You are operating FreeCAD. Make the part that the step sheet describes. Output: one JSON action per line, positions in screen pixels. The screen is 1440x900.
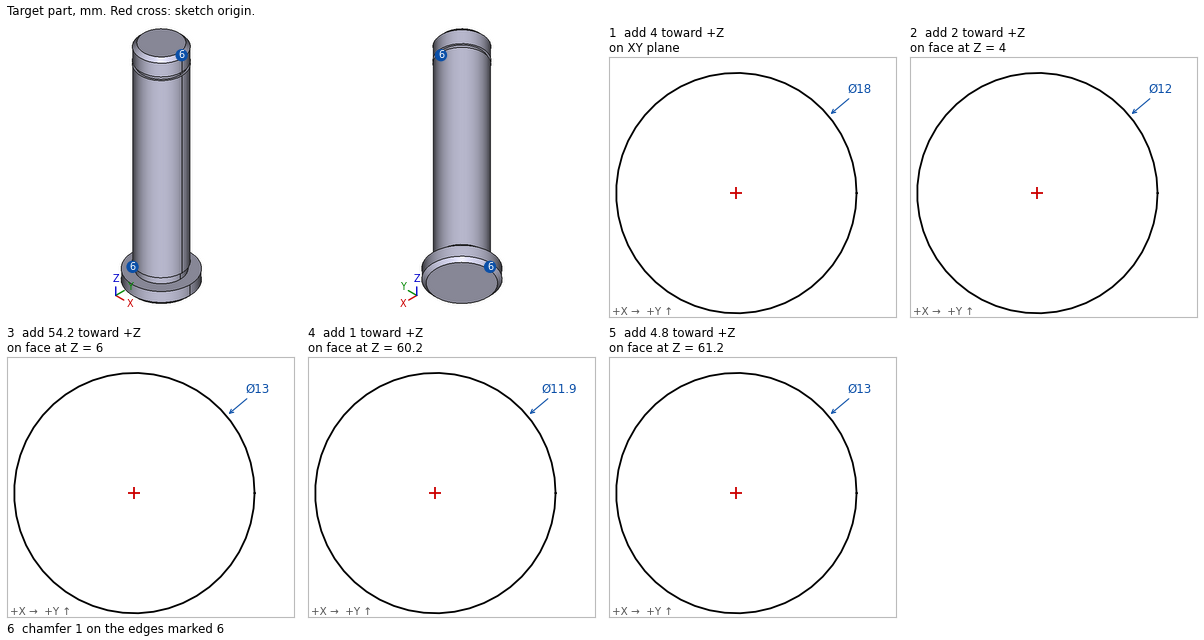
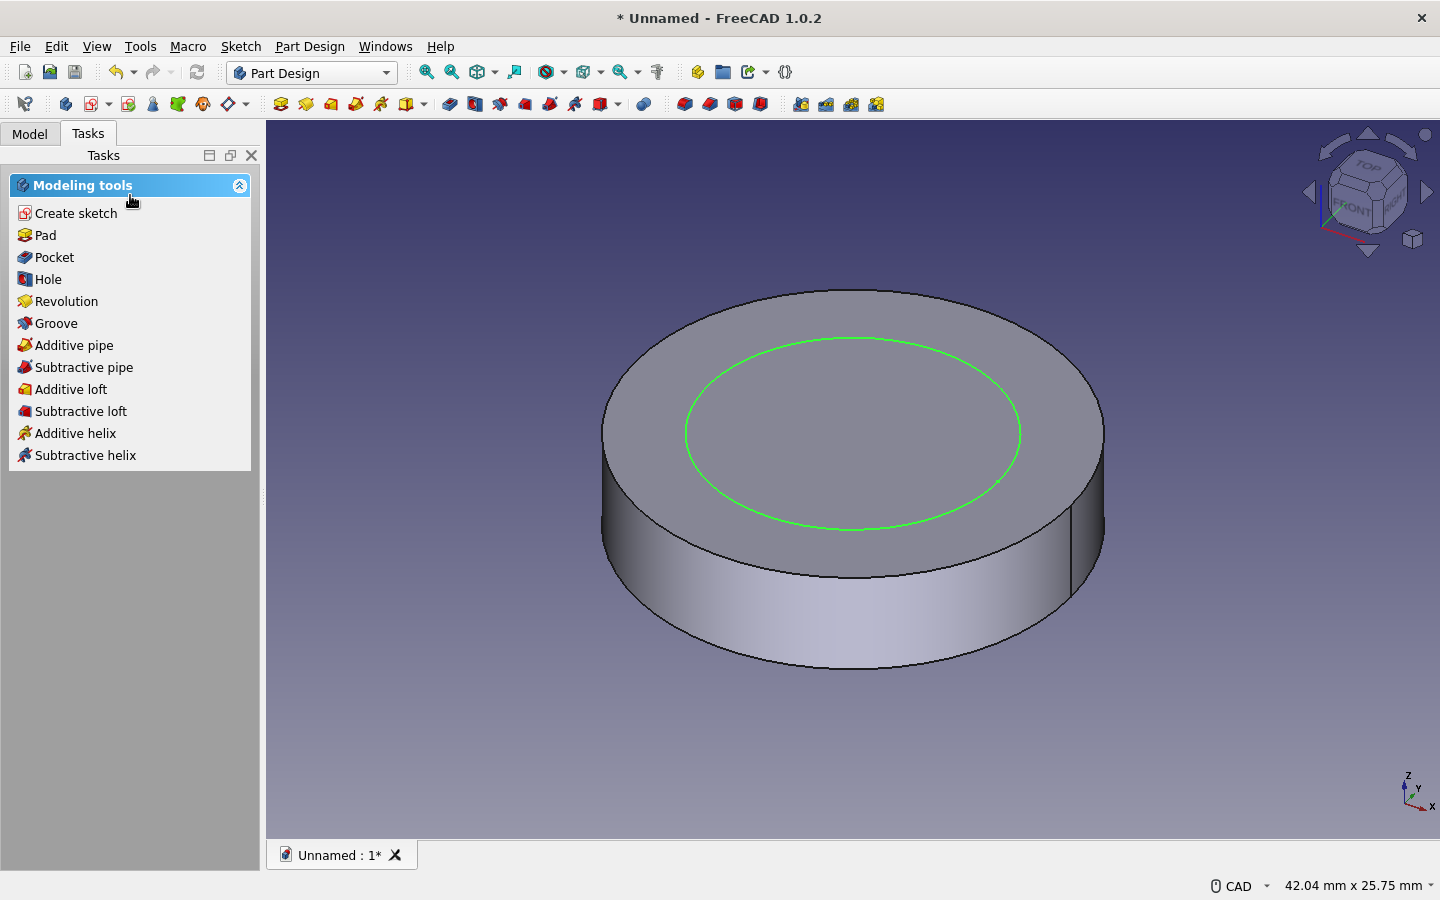
{"action": "left_click", "coordinate": [281, 104]}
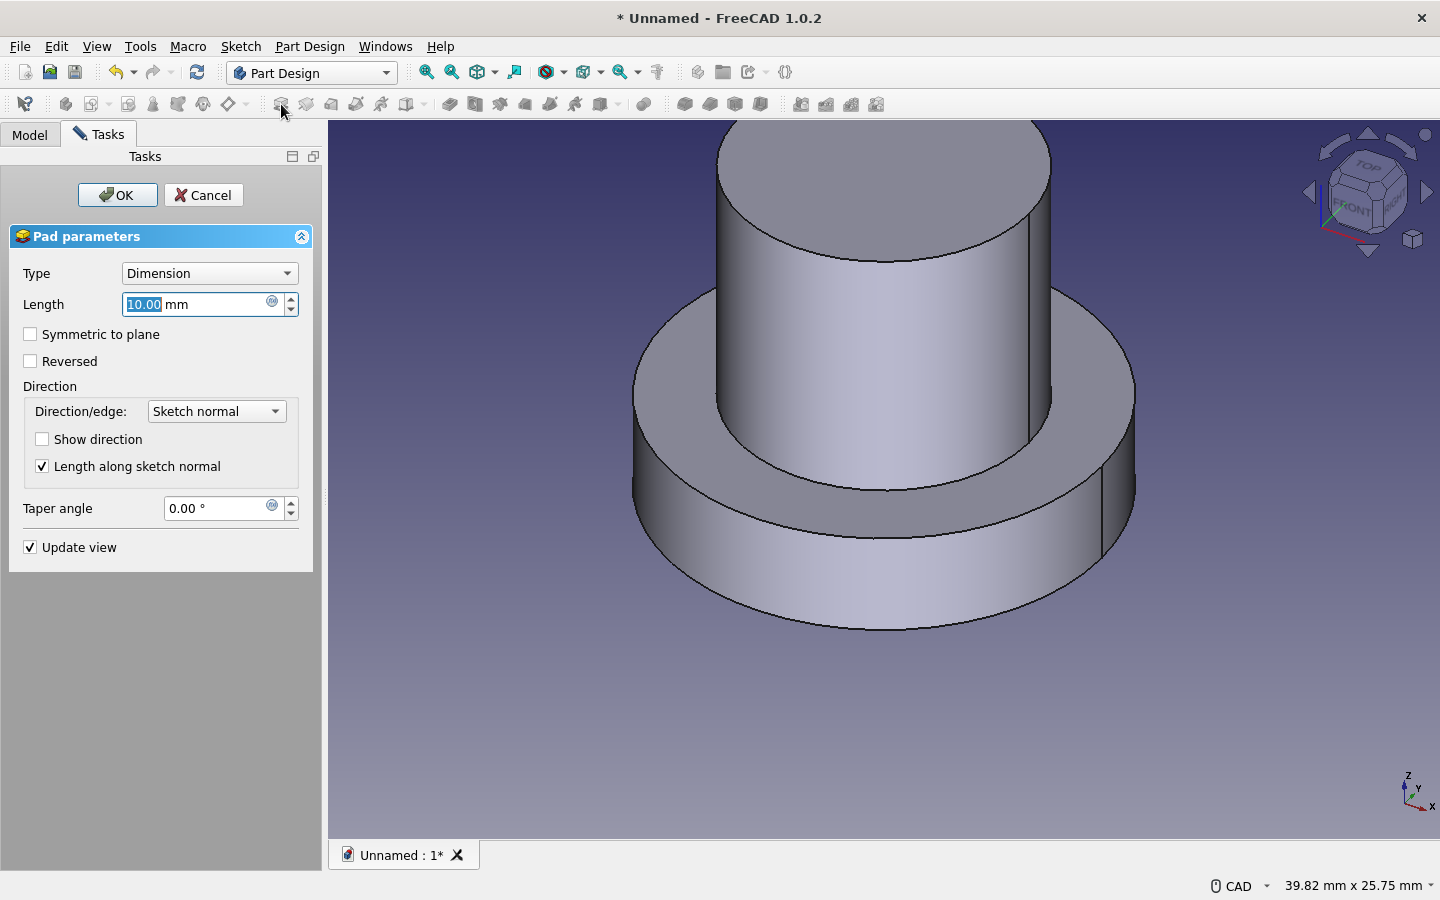
{"action": "type", "text": "2"}
{"action": "key", "text": "Tab"}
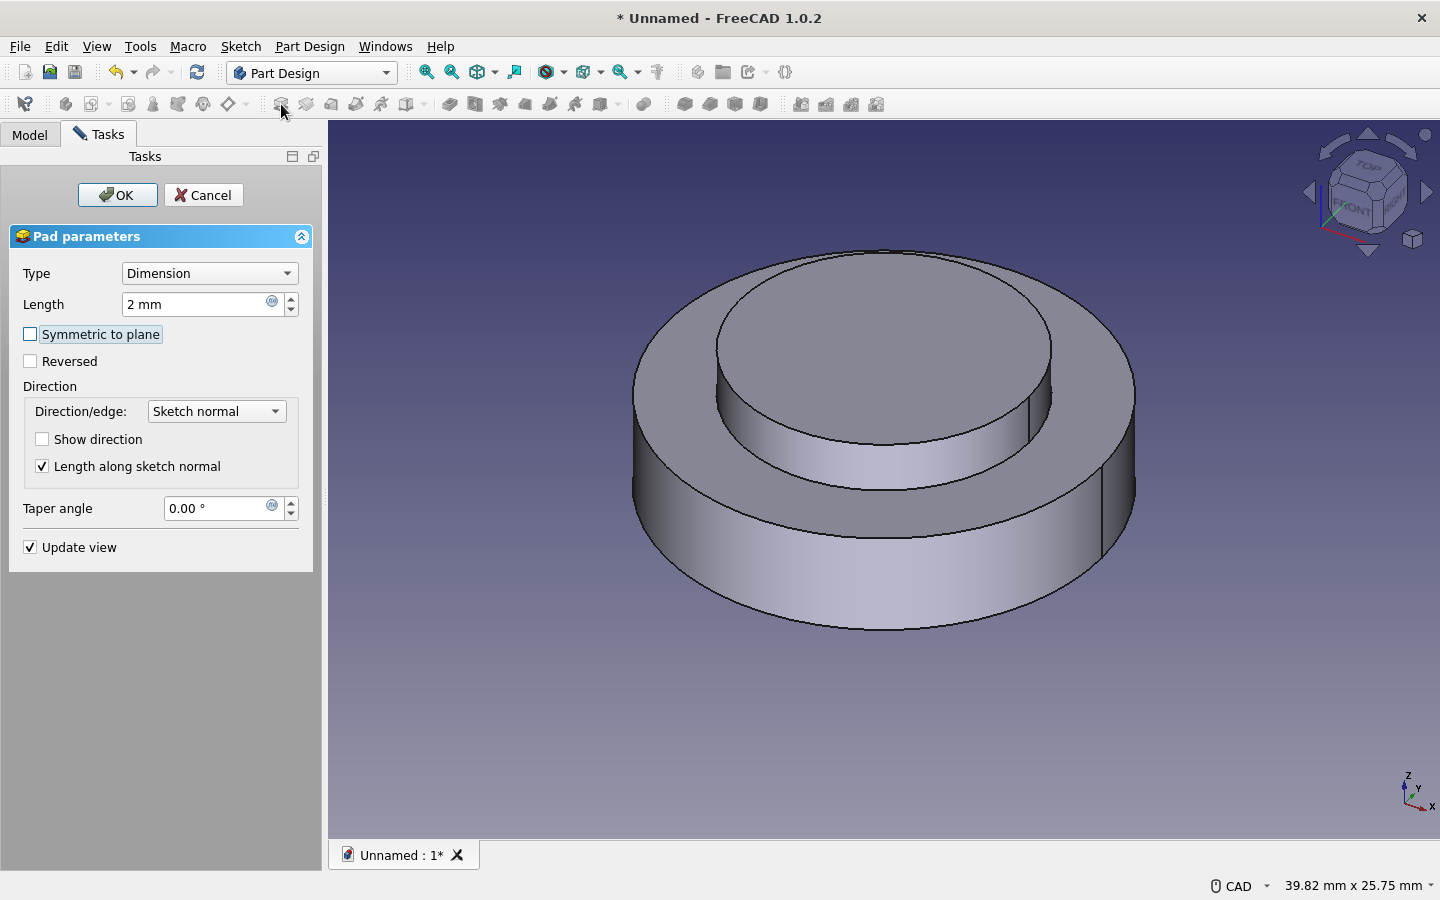
{"action": "left_click", "coordinate": [118, 195]}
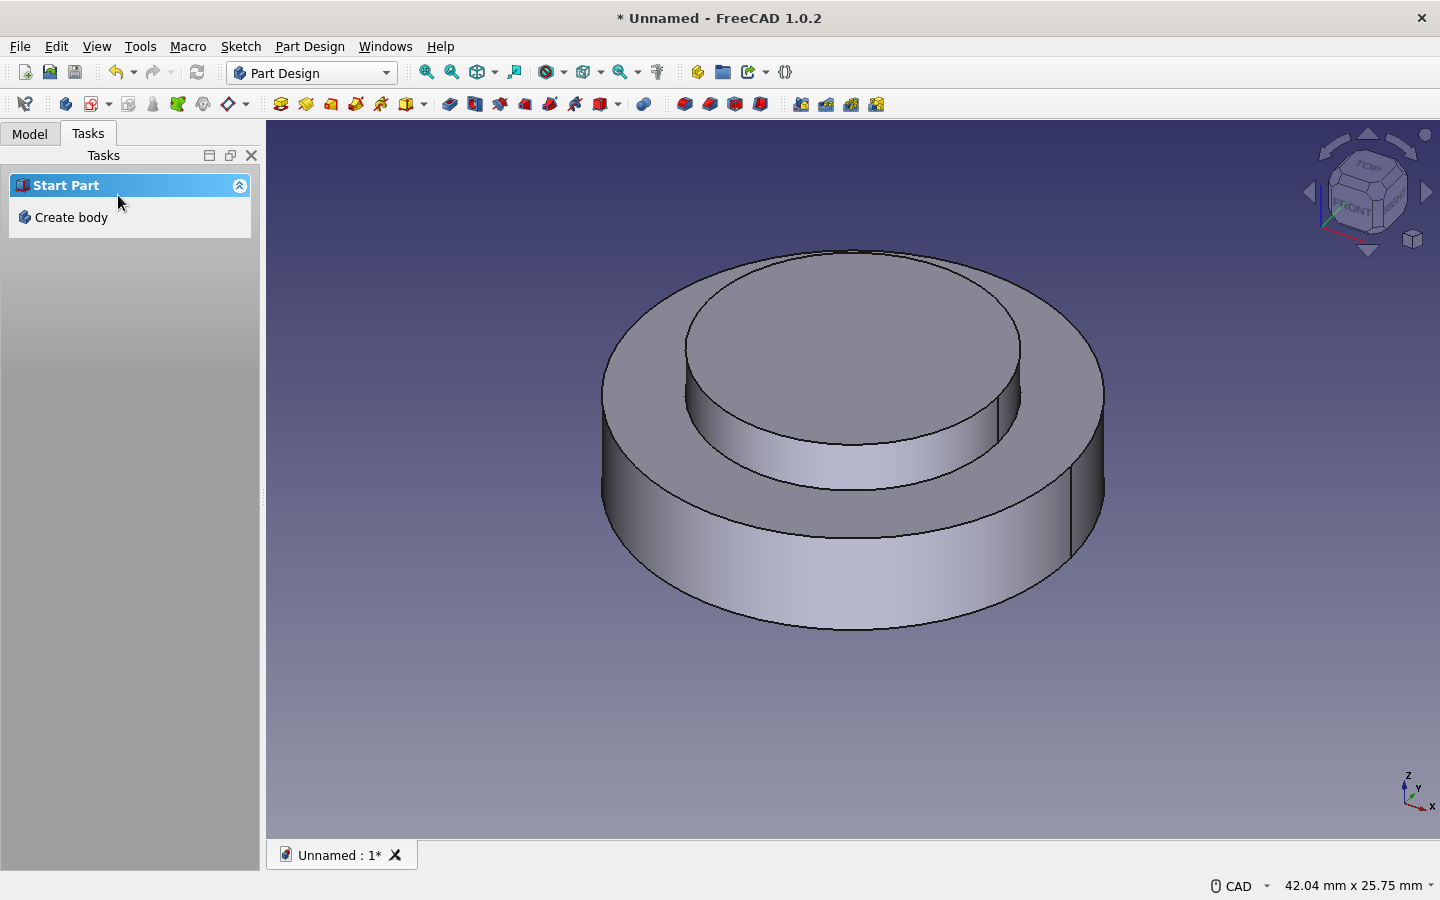
{"action": "left_click", "coordinate": [853, 348]}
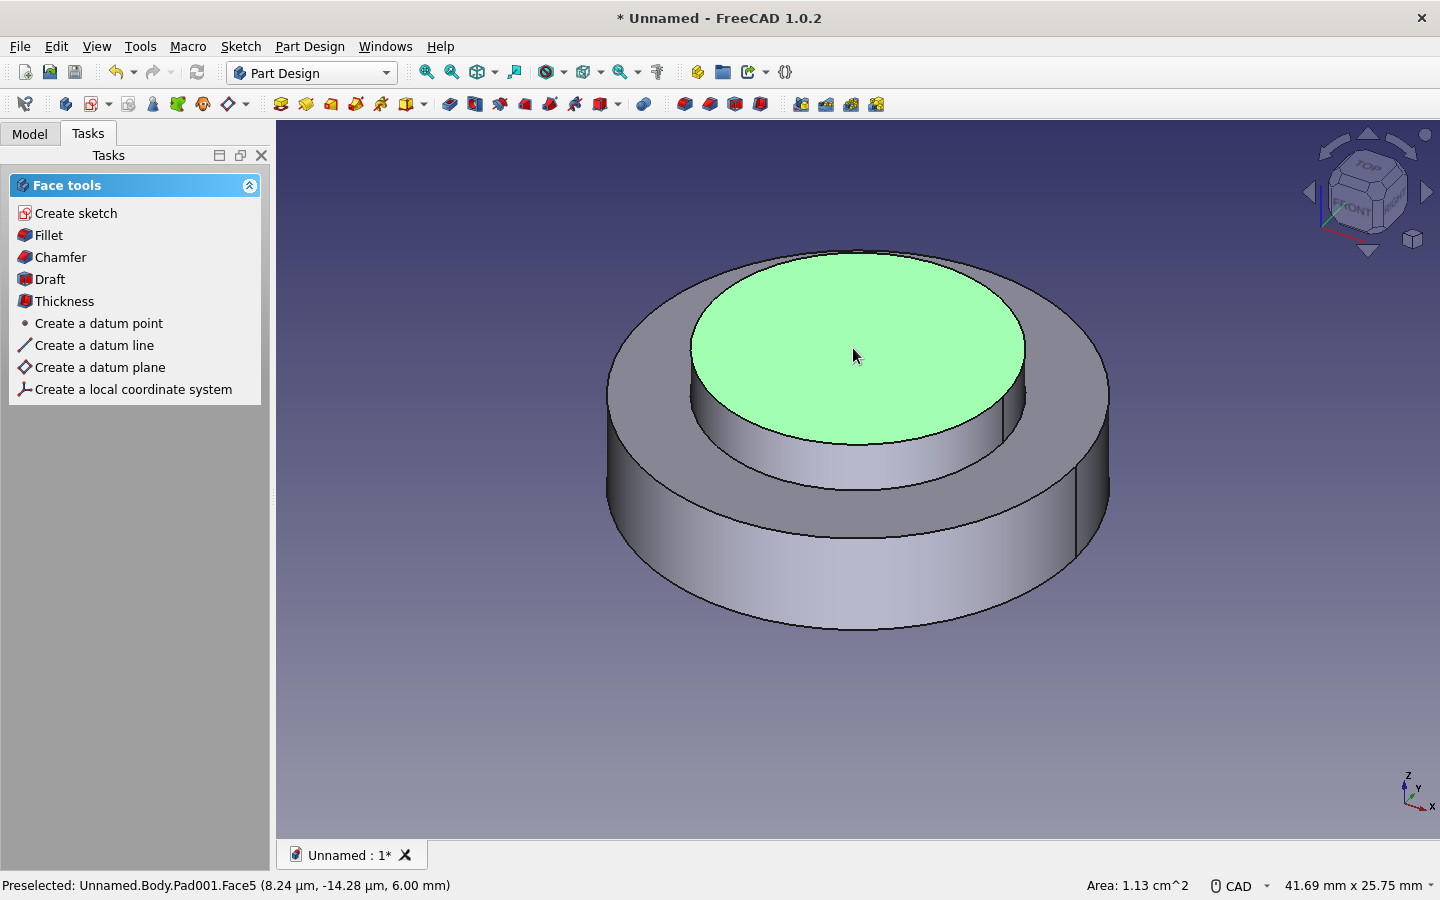
{"action": "left_click", "coordinate": [90, 104]}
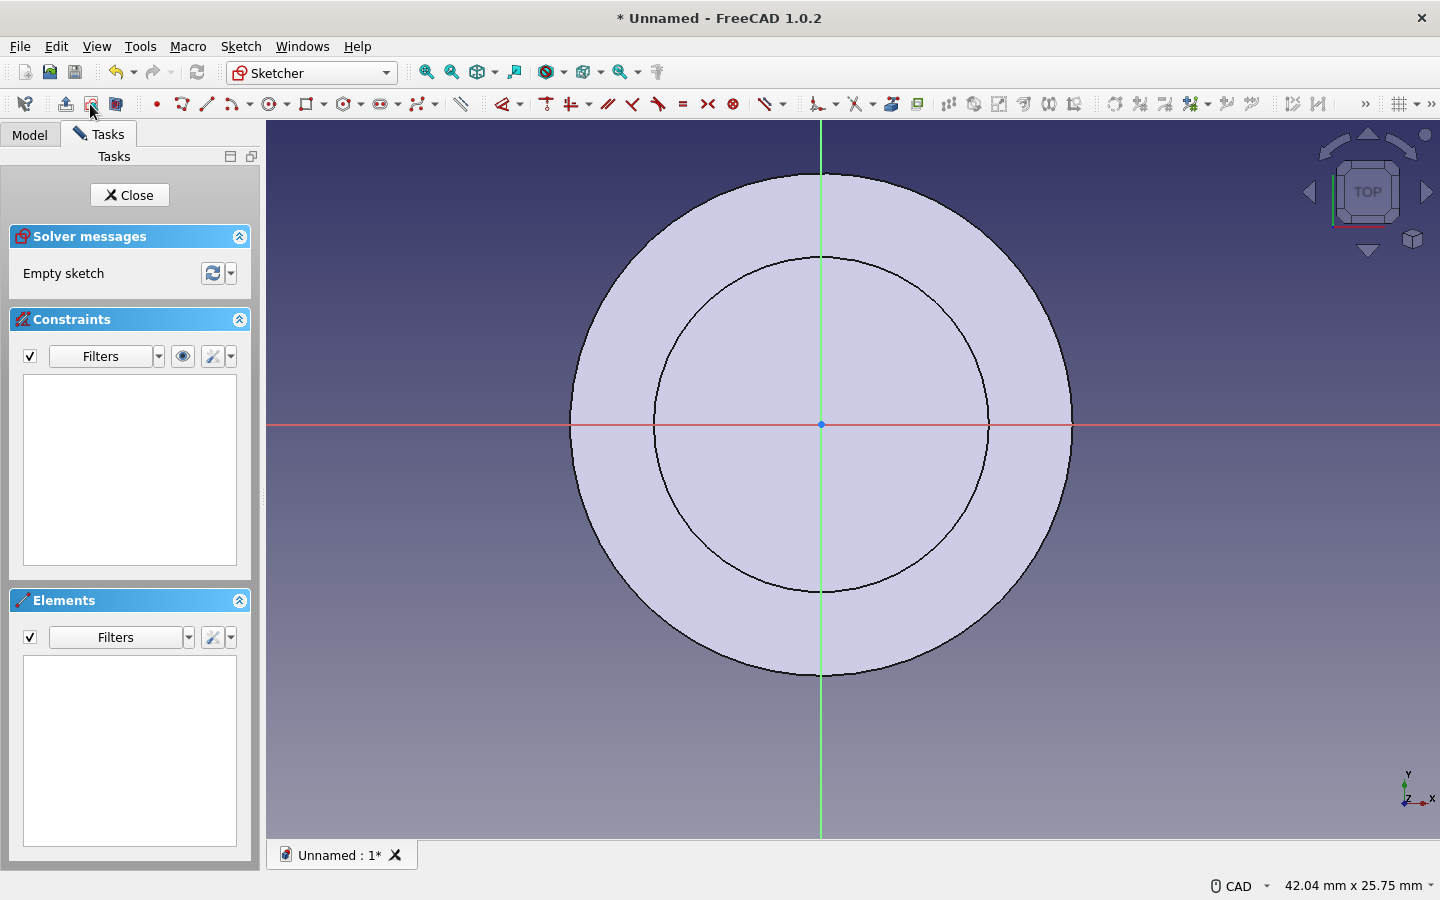
{"action": "left_click", "coordinate": [268, 104]}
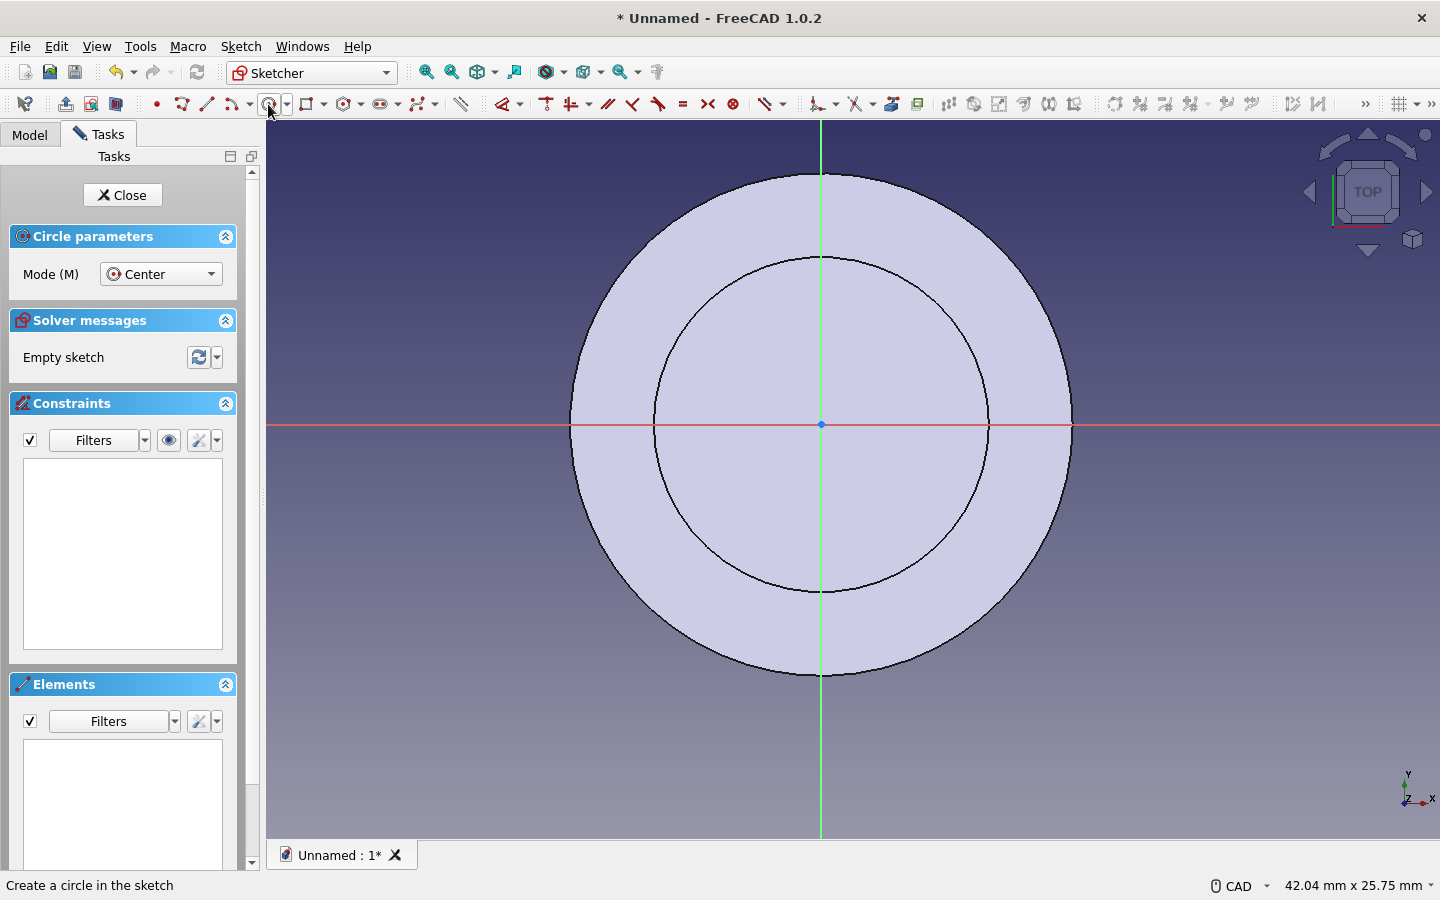
{"action": "left_click", "coordinate": [821, 425]}
{"action": "left_click", "coordinate": [950, 296]}
{"action": "key", "text": "Escape"}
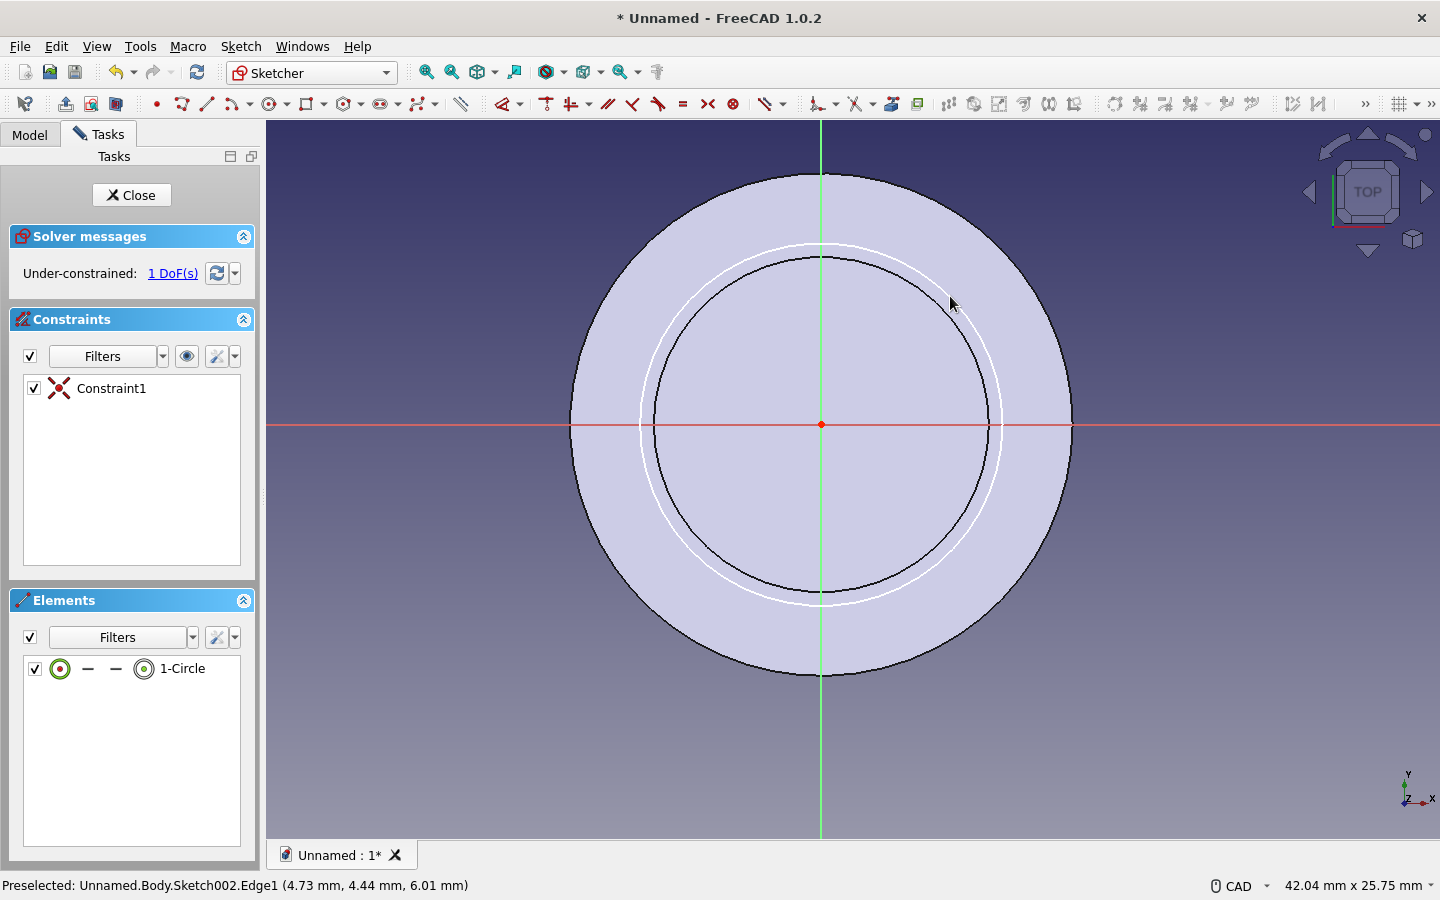
{"action": "left_click", "coordinate": [502, 104]}